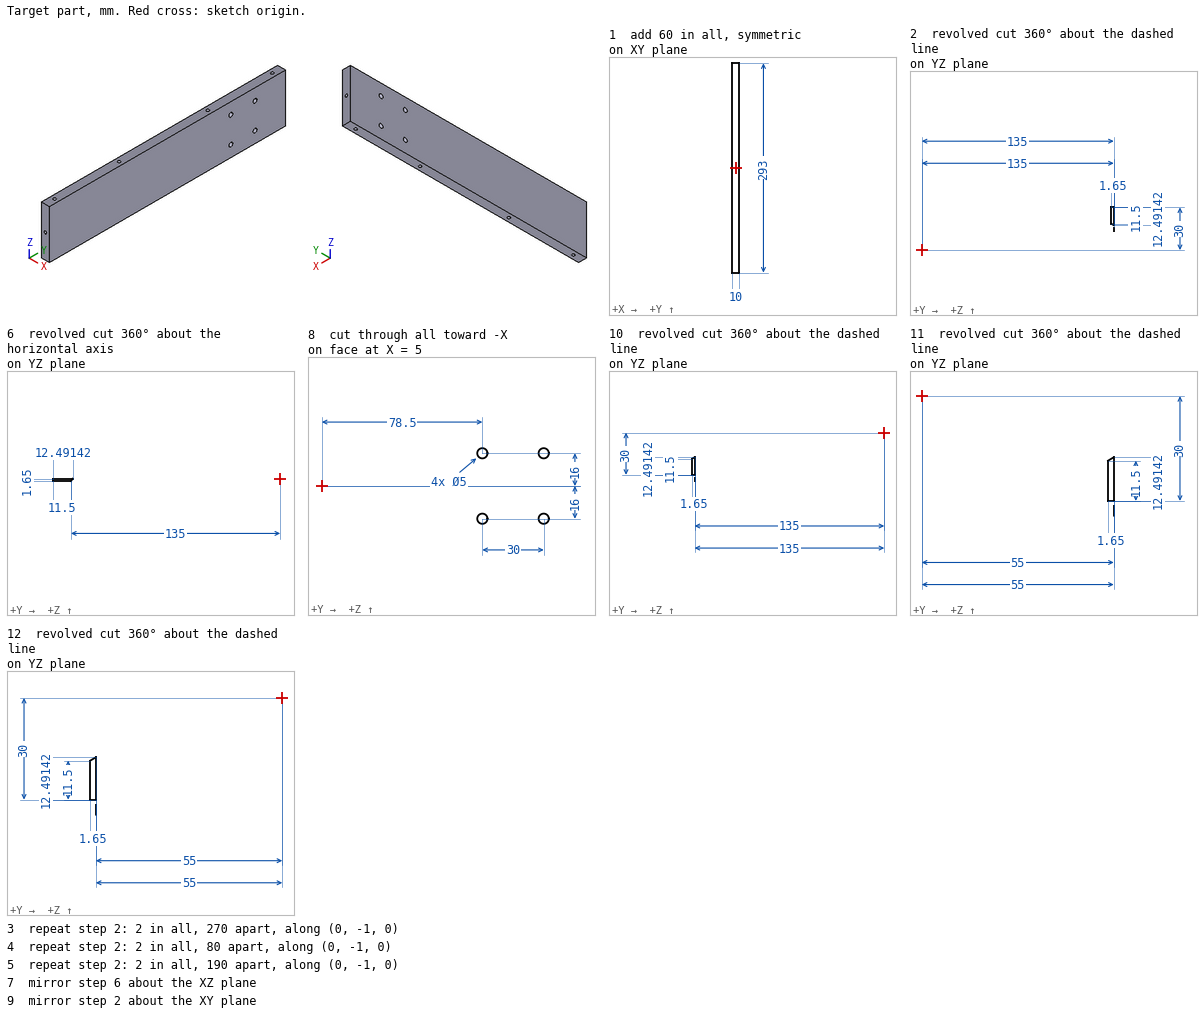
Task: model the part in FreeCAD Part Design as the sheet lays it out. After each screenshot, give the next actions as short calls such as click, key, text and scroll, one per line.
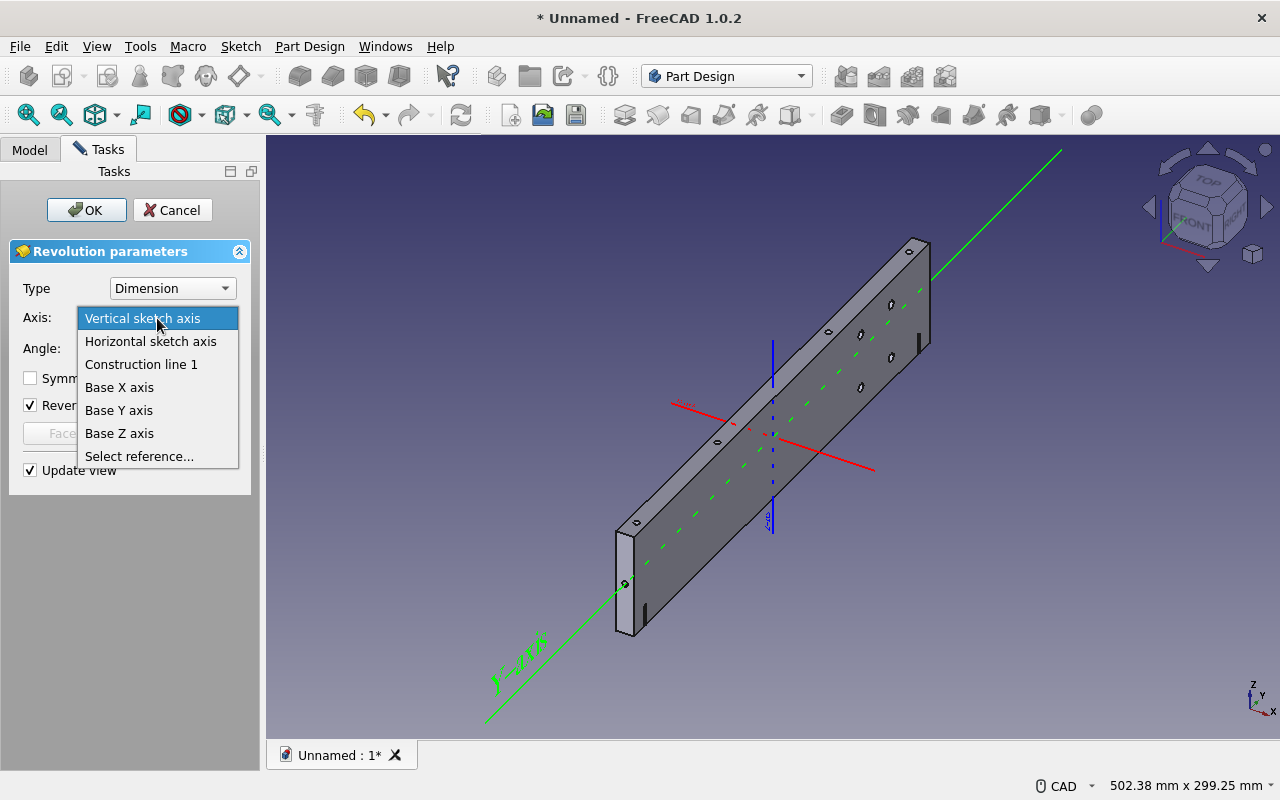
click(156, 364)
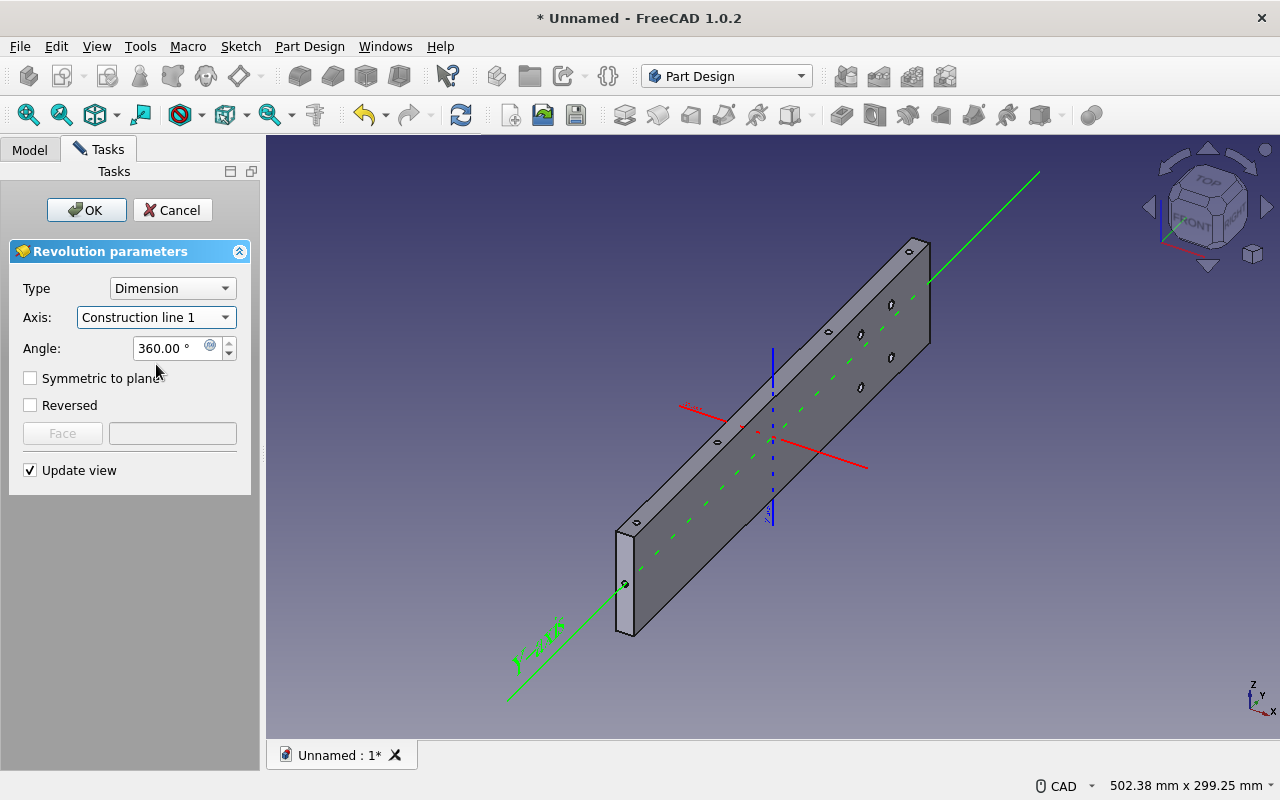
click(87, 210)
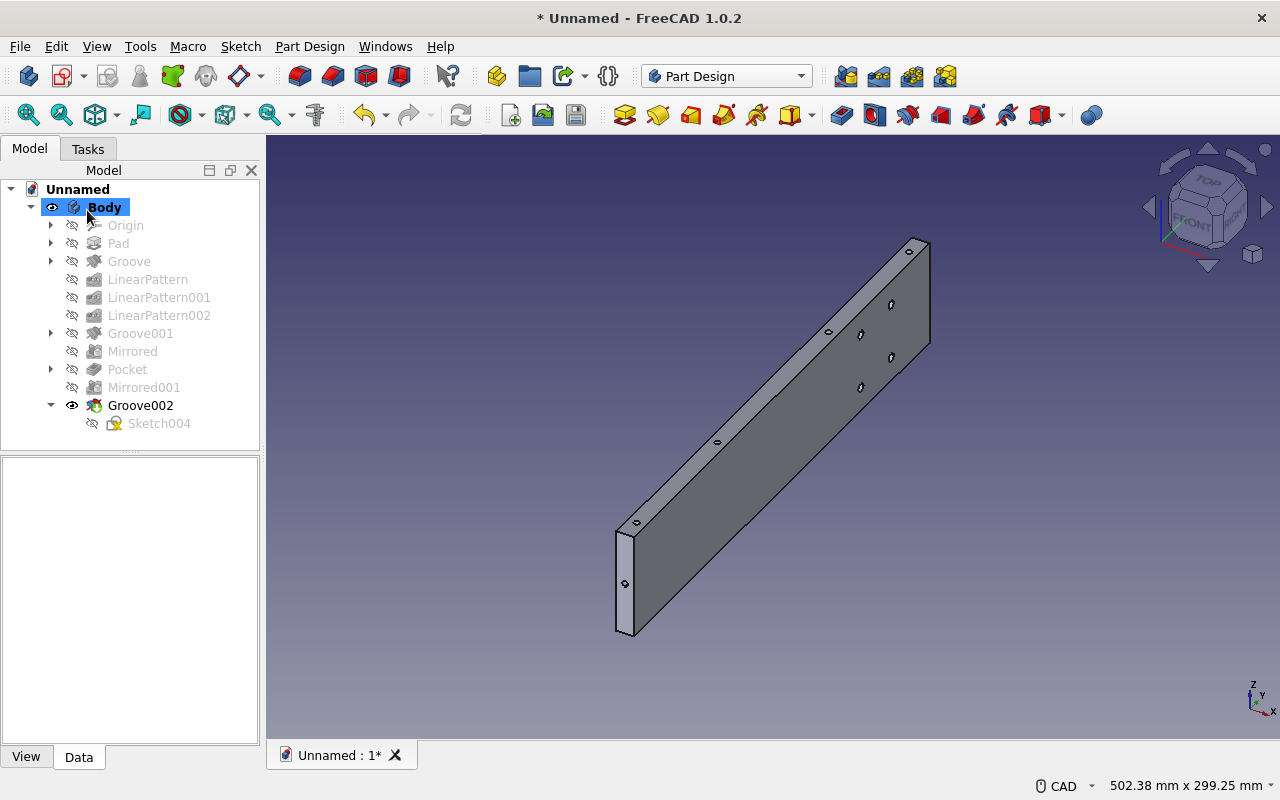
click(62, 76)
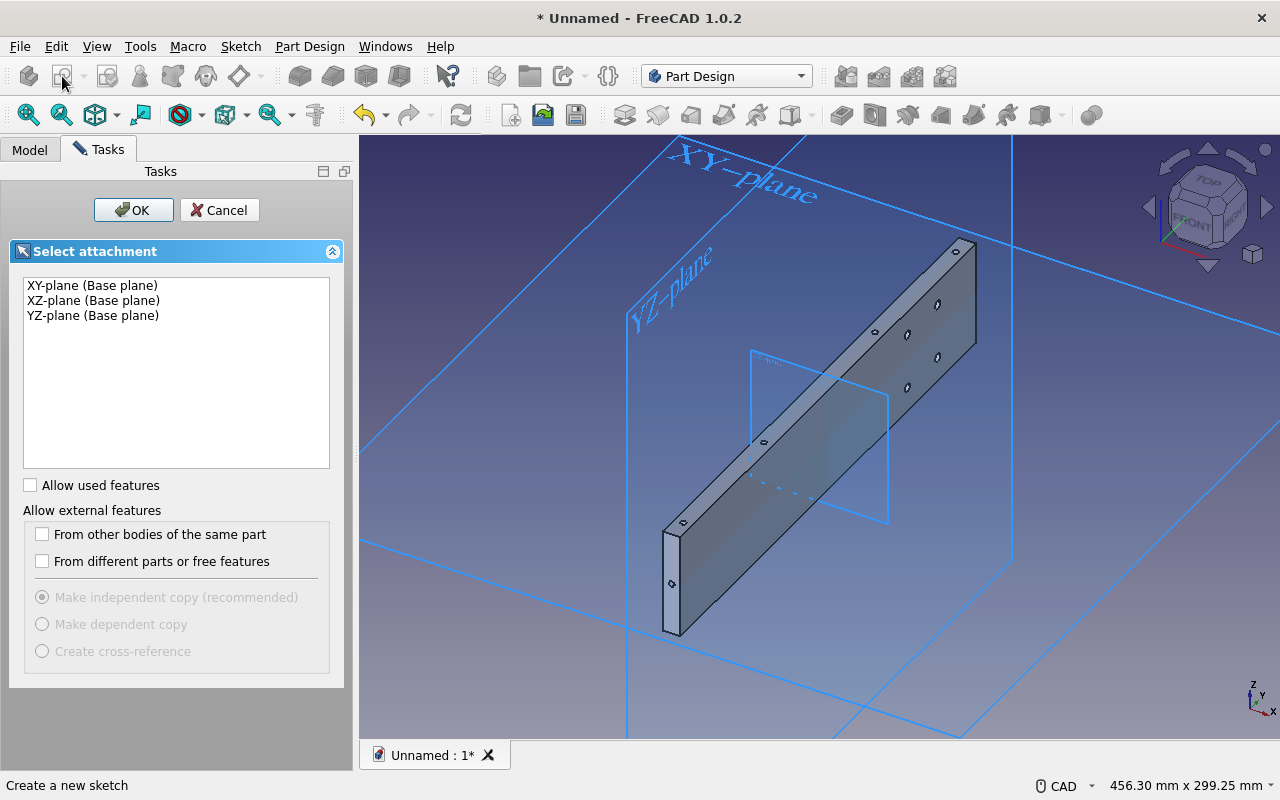
click(84, 316)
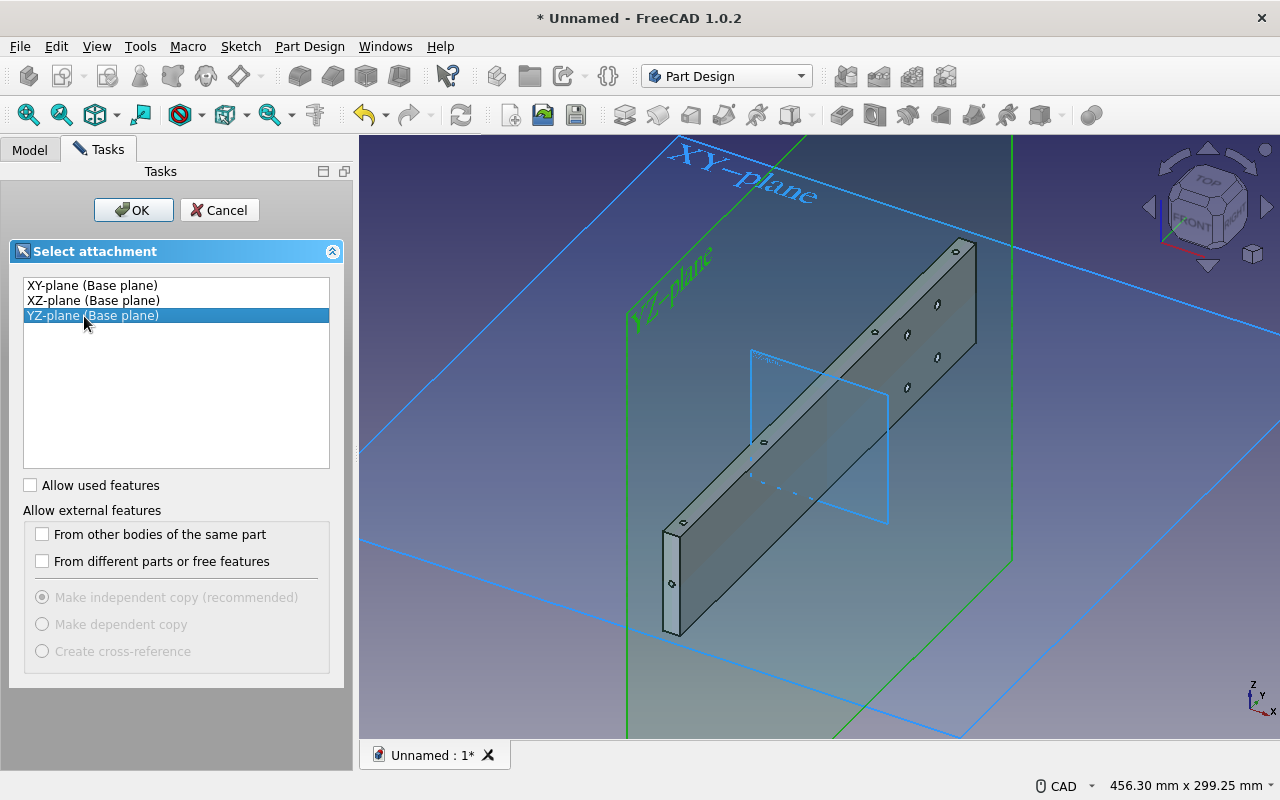
click(134, 210)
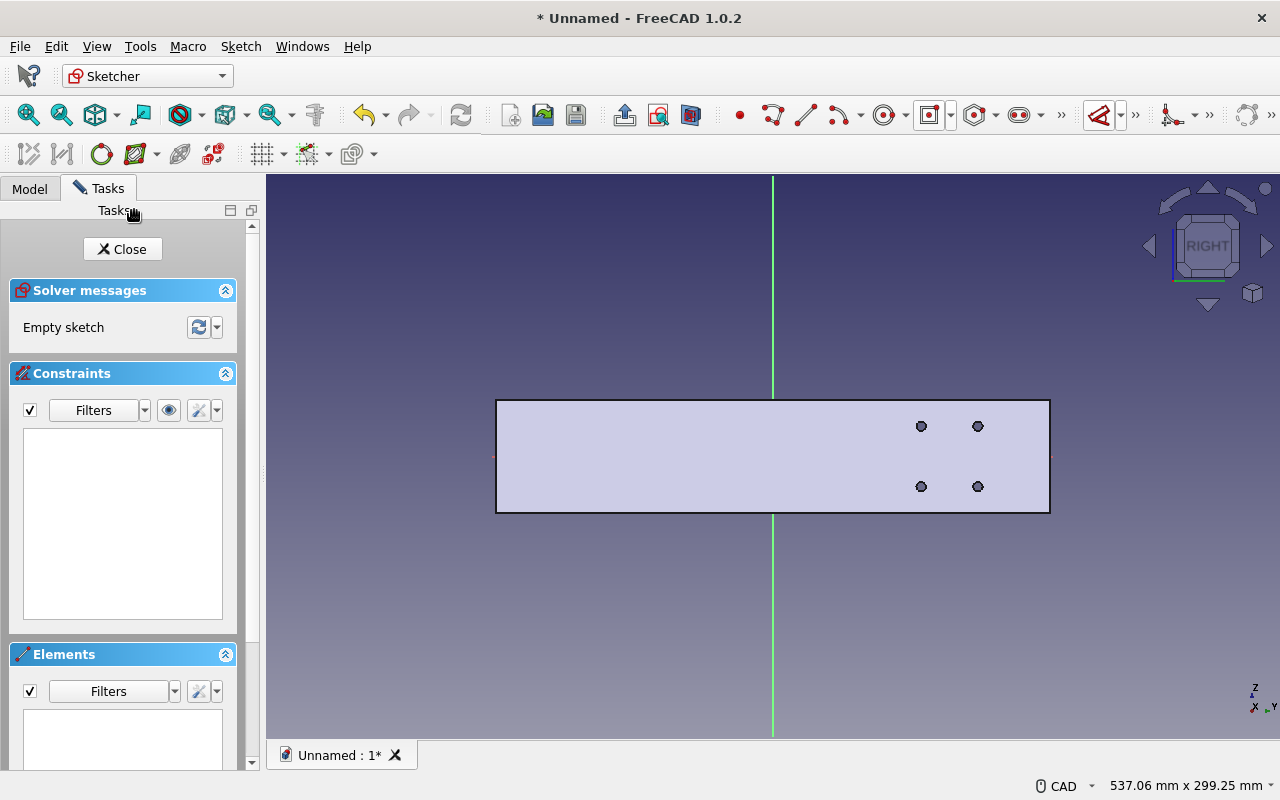
click(691, 116)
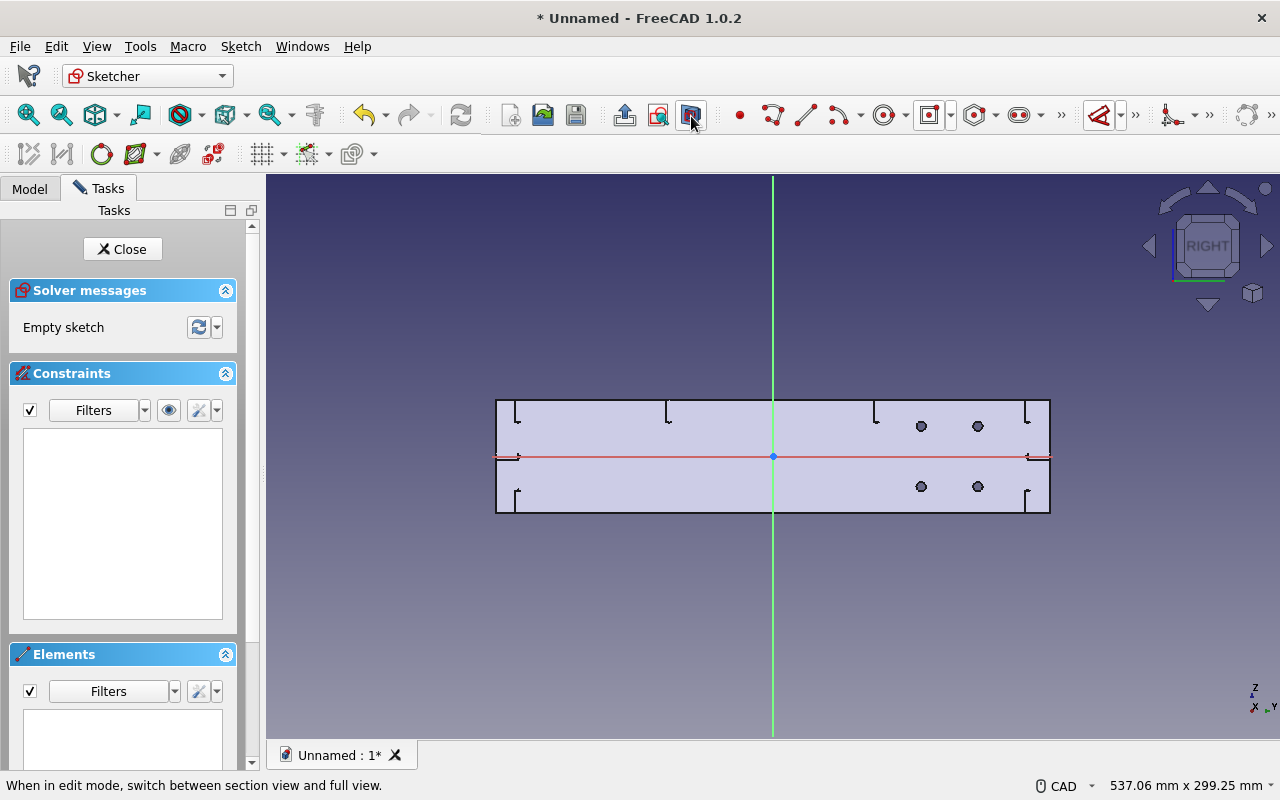
scroll(892, 511, up, 12)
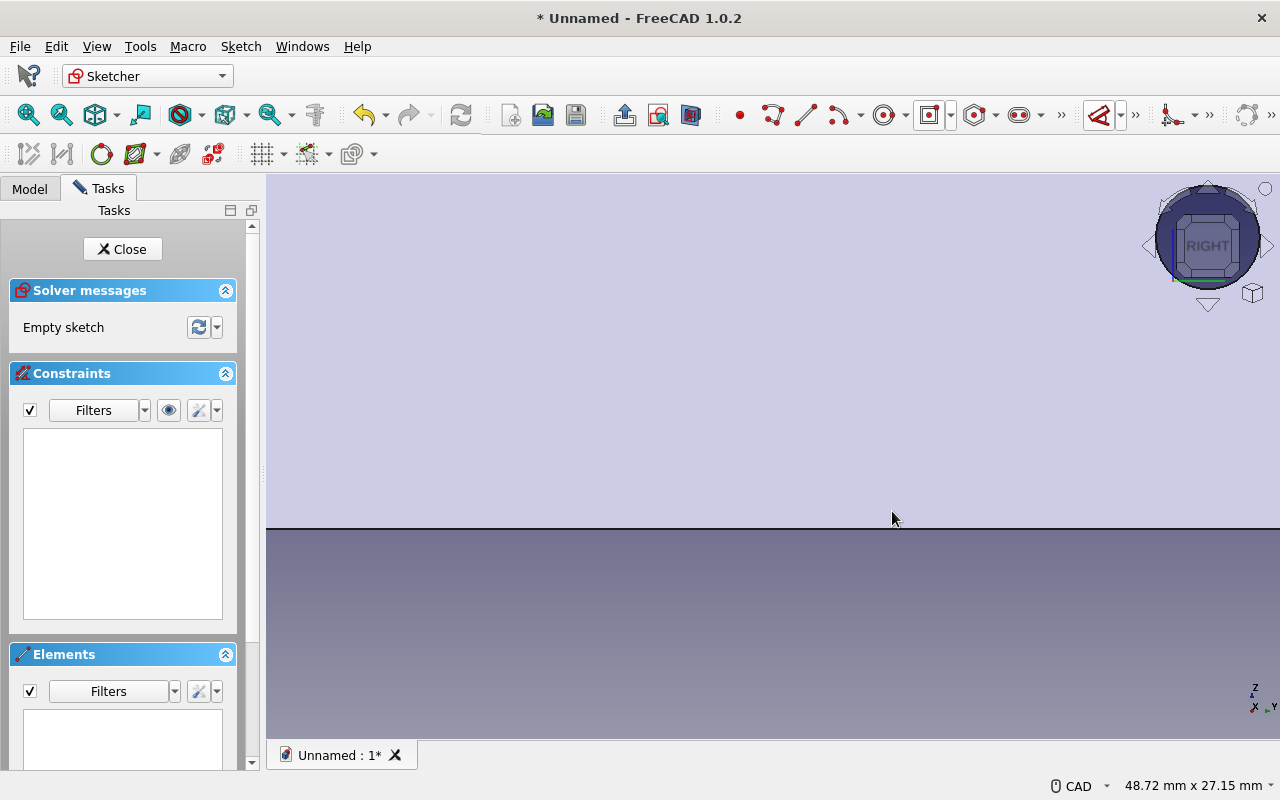
click(773, 116)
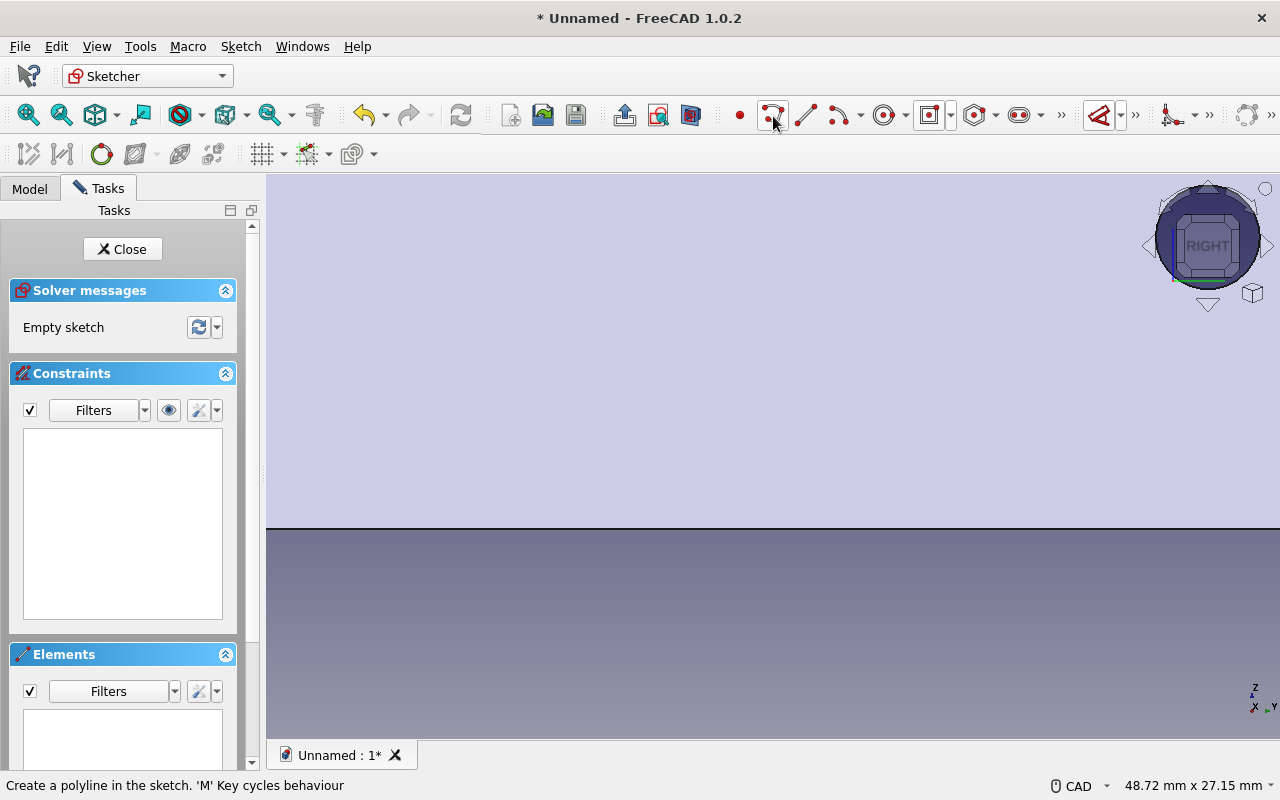
click(684, 289)
click(684, 529)
click(719, 529)
click(719, 269)
click(684, 290)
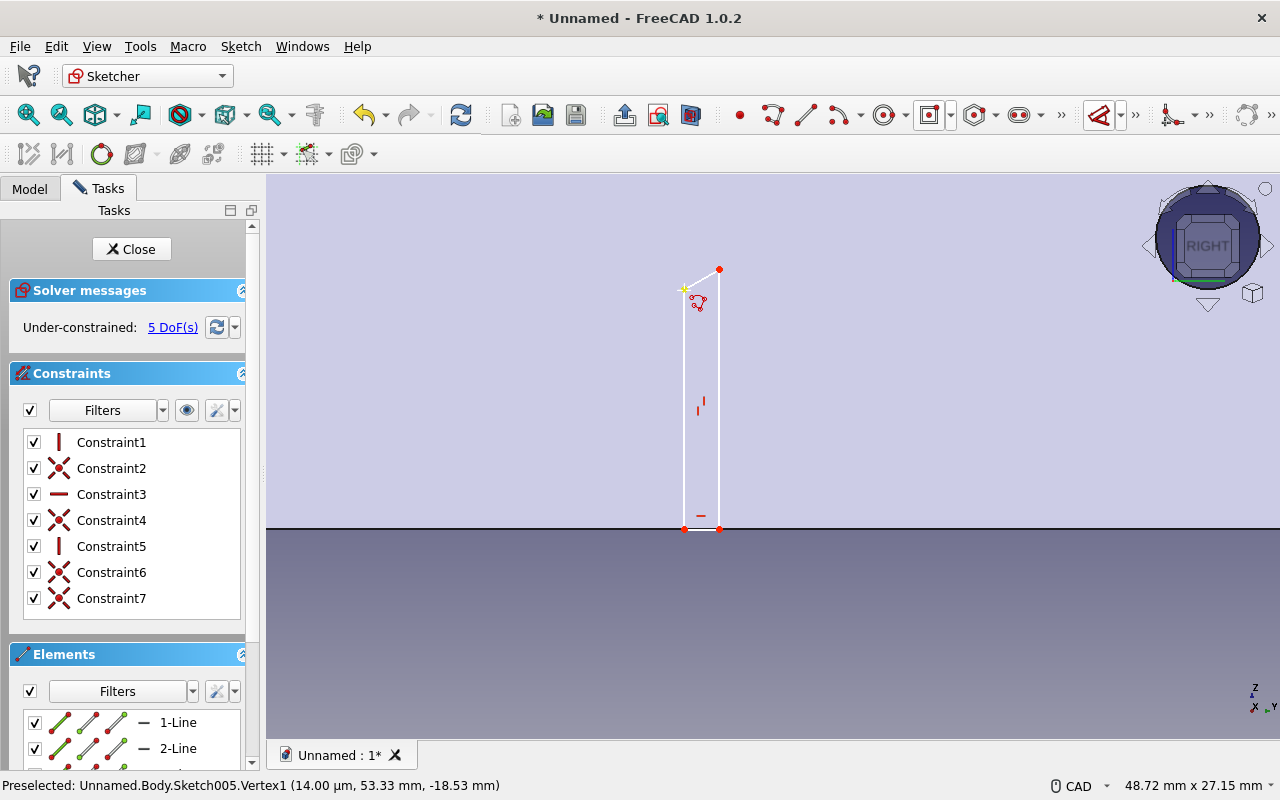
click(806, 116)